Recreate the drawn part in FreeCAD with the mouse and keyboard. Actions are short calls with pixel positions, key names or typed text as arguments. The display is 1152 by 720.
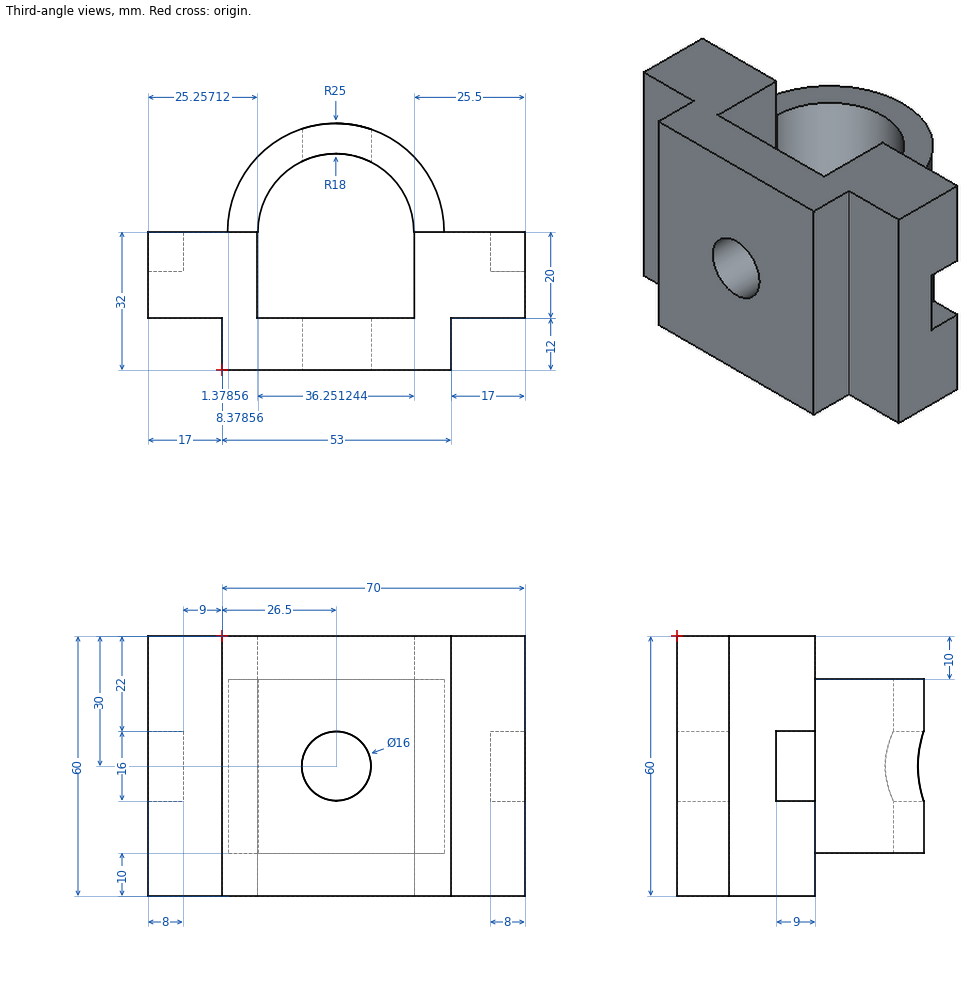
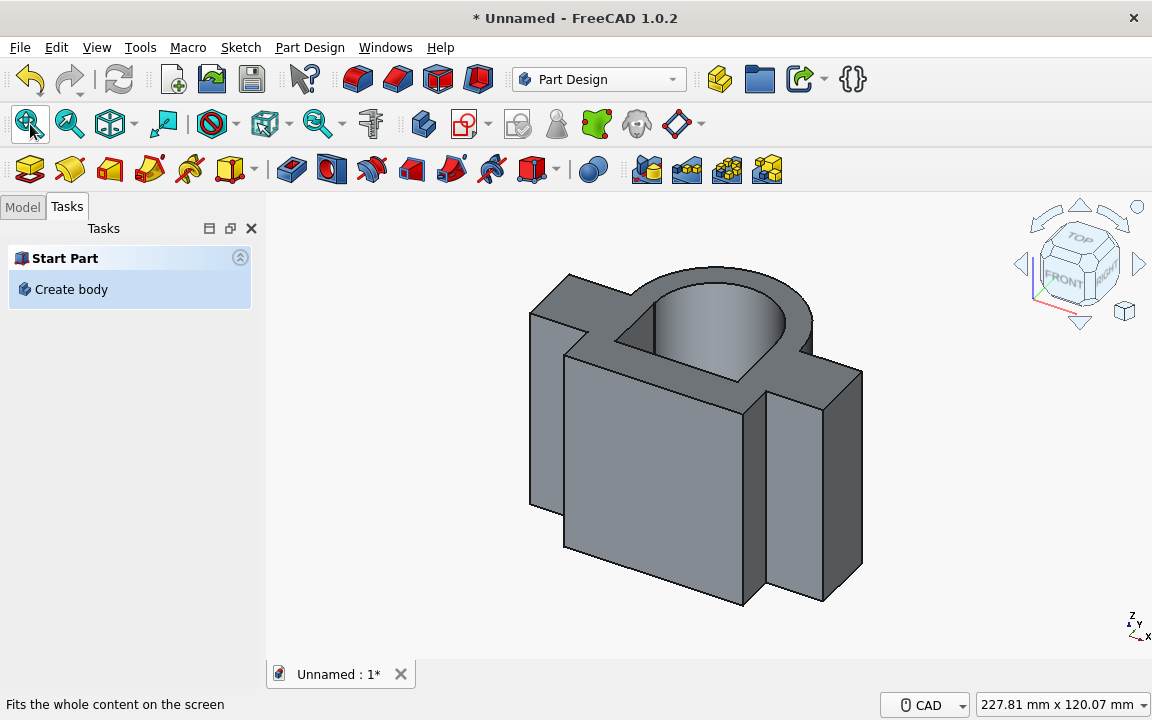
click(464, 124)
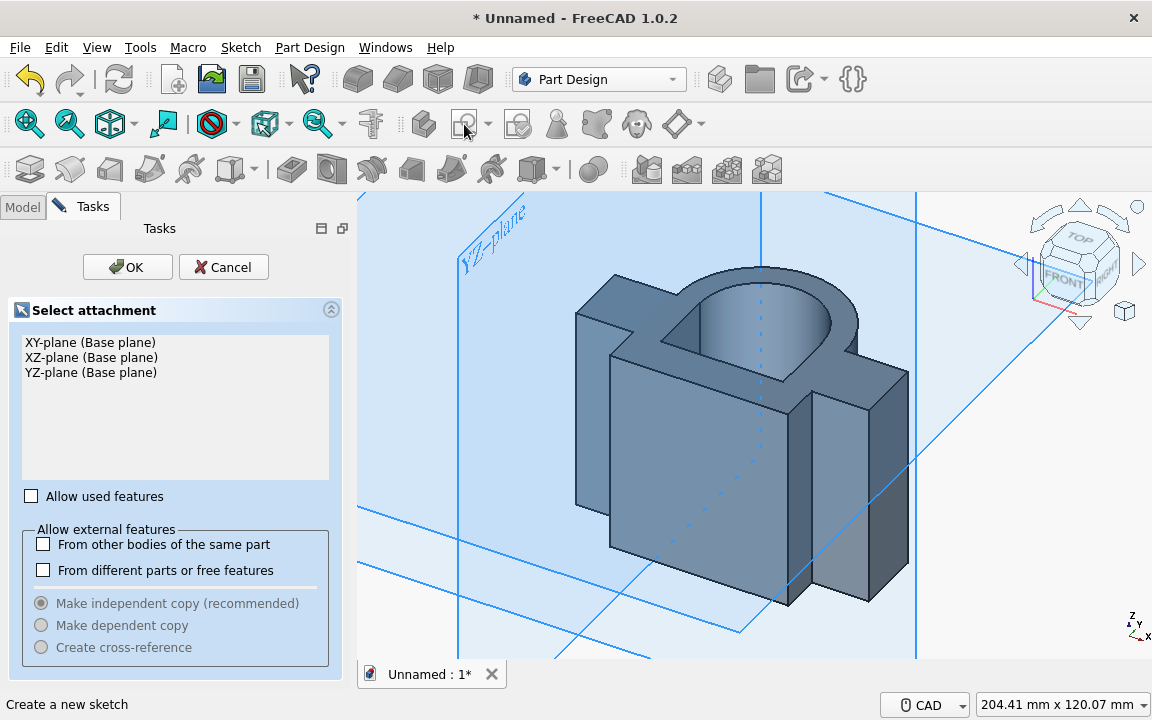
click(82, 342)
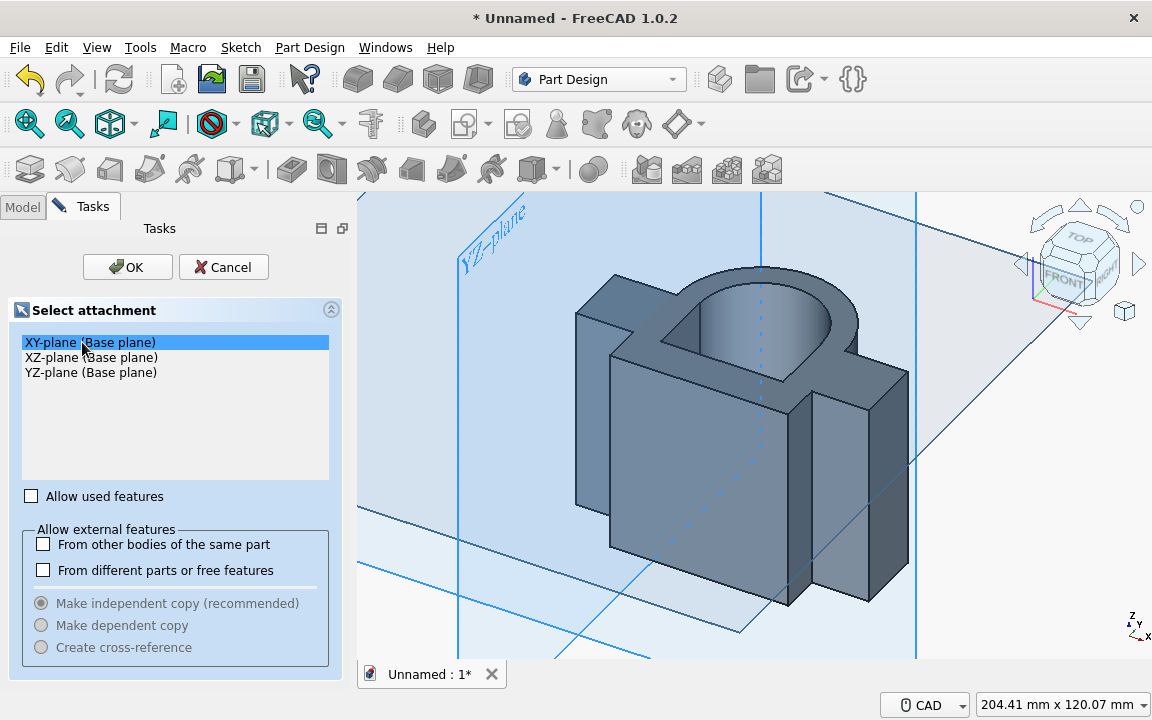
click(128, 267)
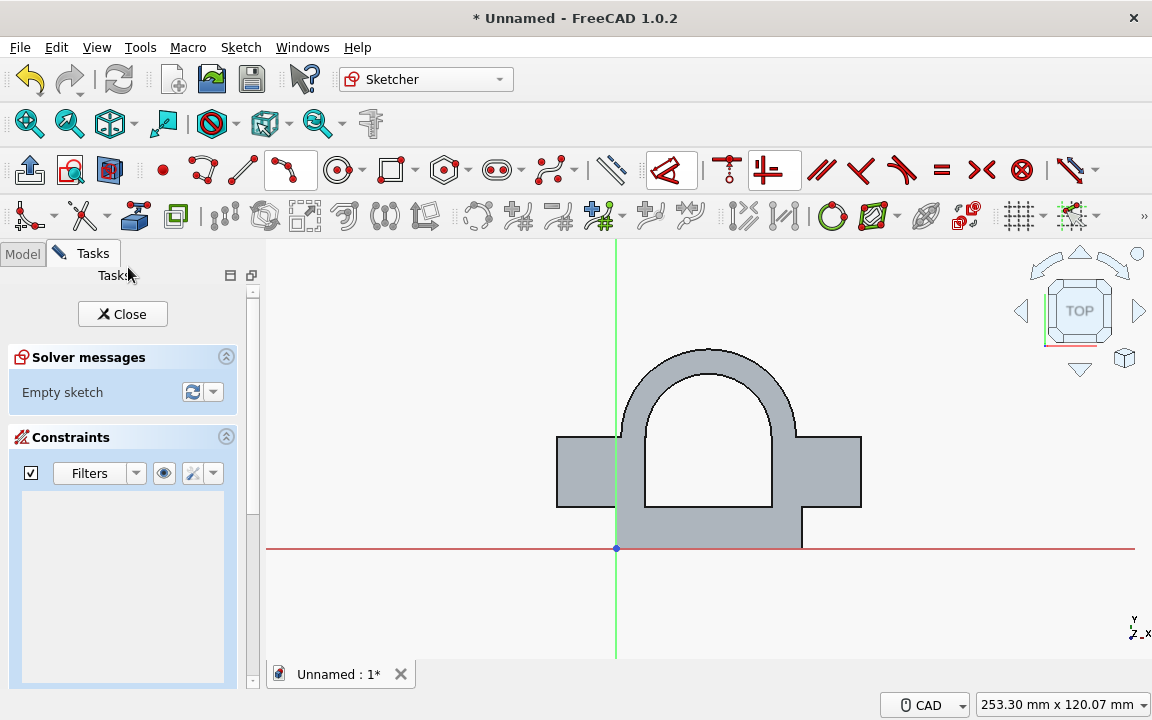
click(244, 170)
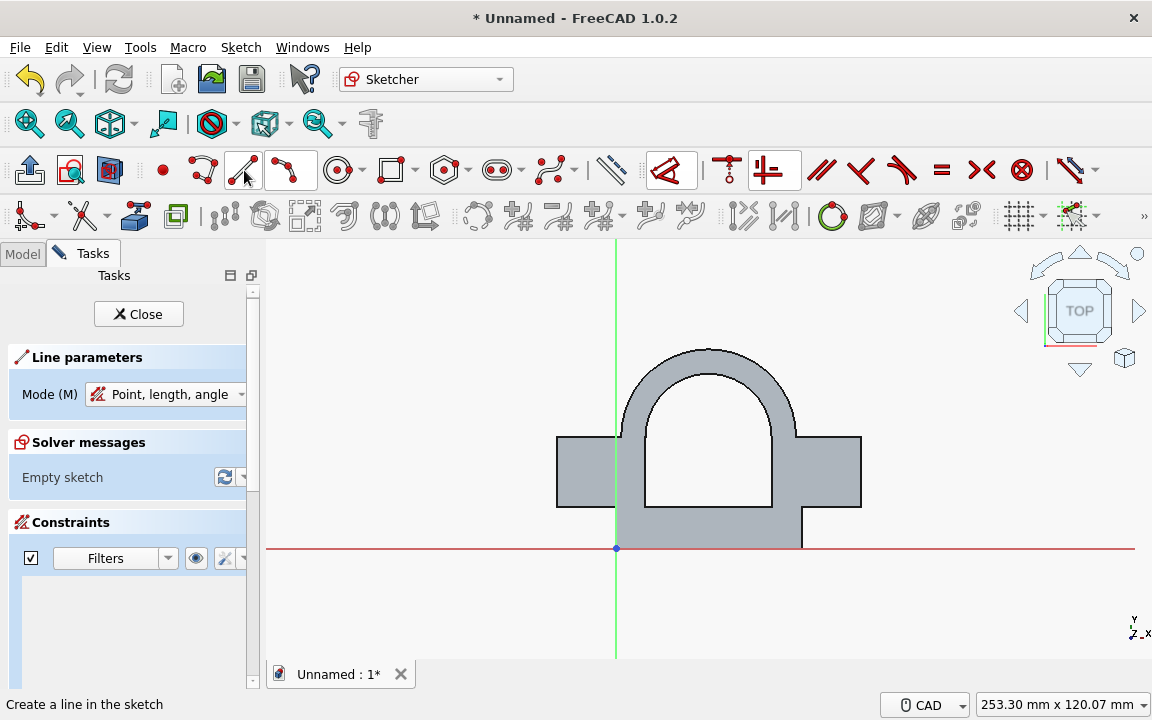
scroll(621, 437, up, 6)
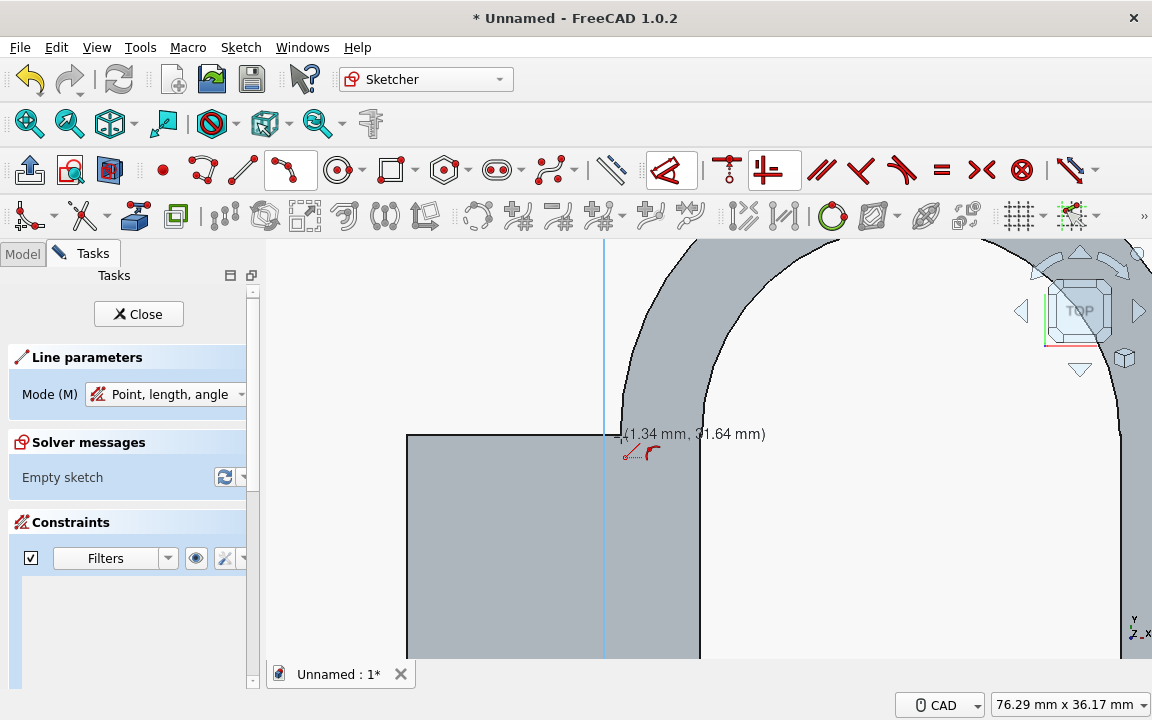
click(621, 435)
click(702, 435)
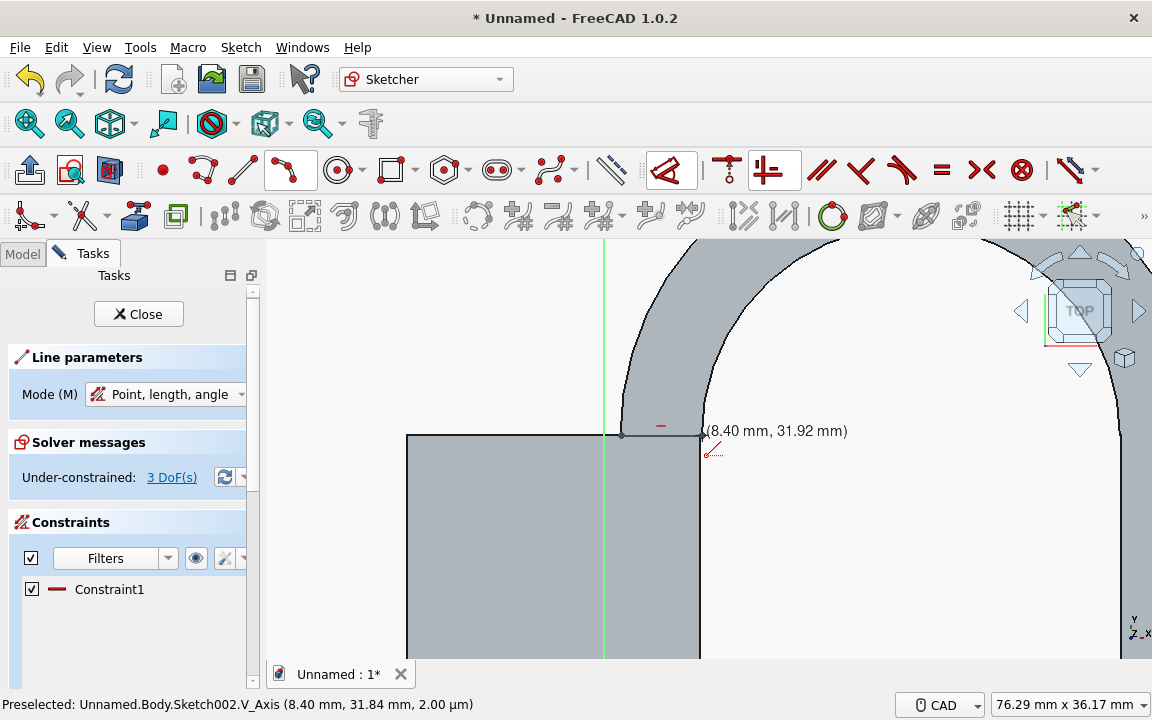
scroll(488, 433, down, 5)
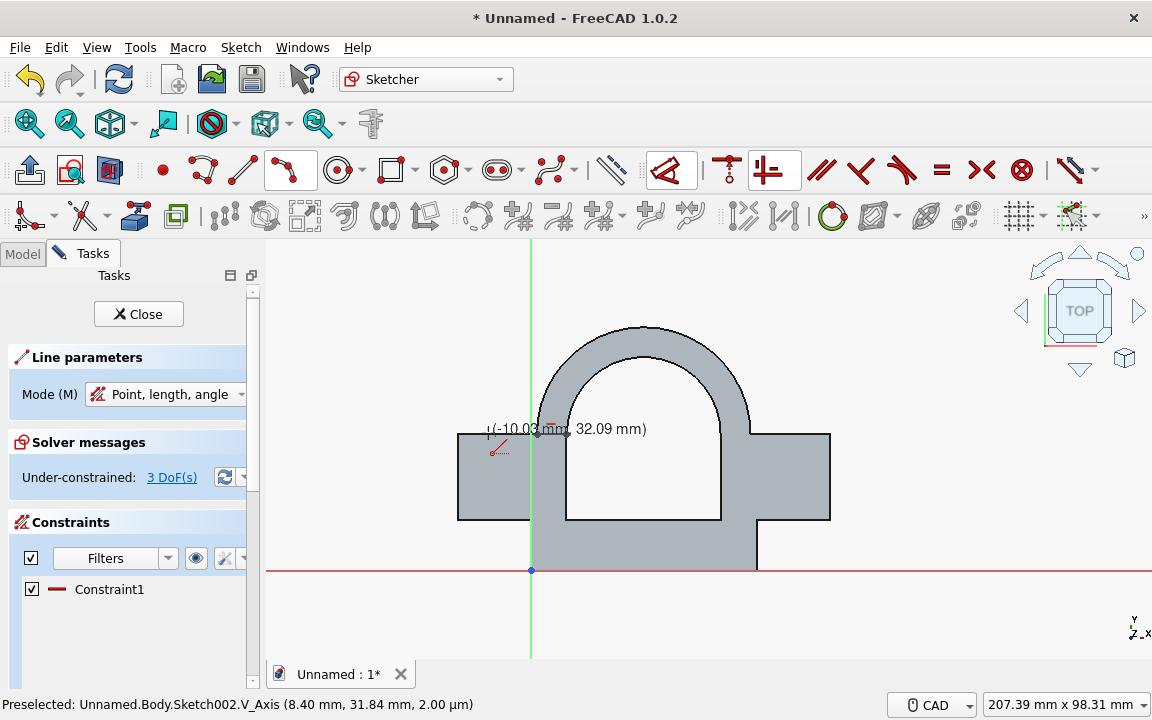
click(721, 434)
click(751, 434)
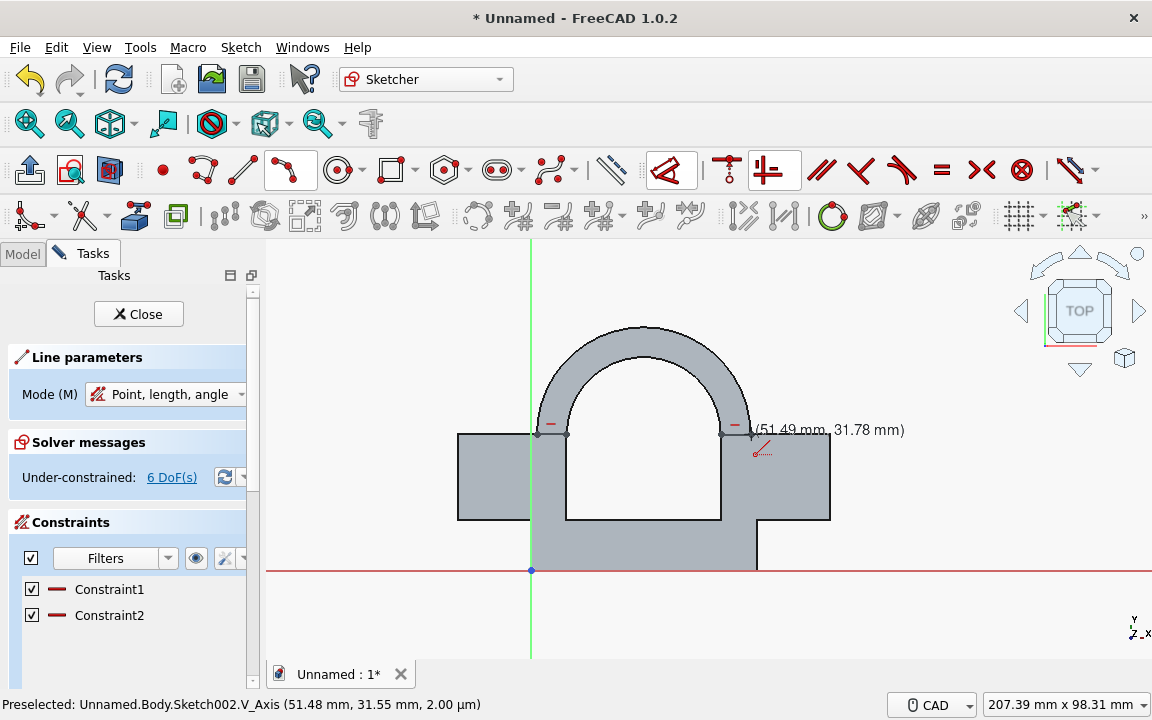
click(284, 170)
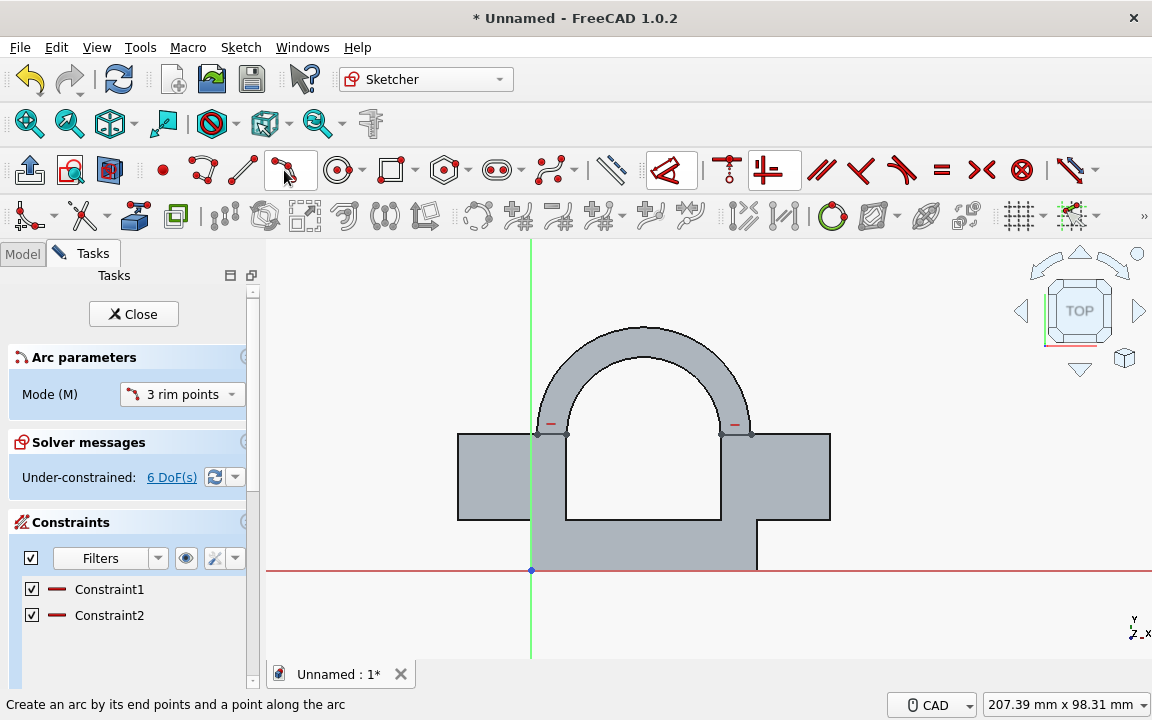
click(567, 434)
click(721, 435)
click(644, 357)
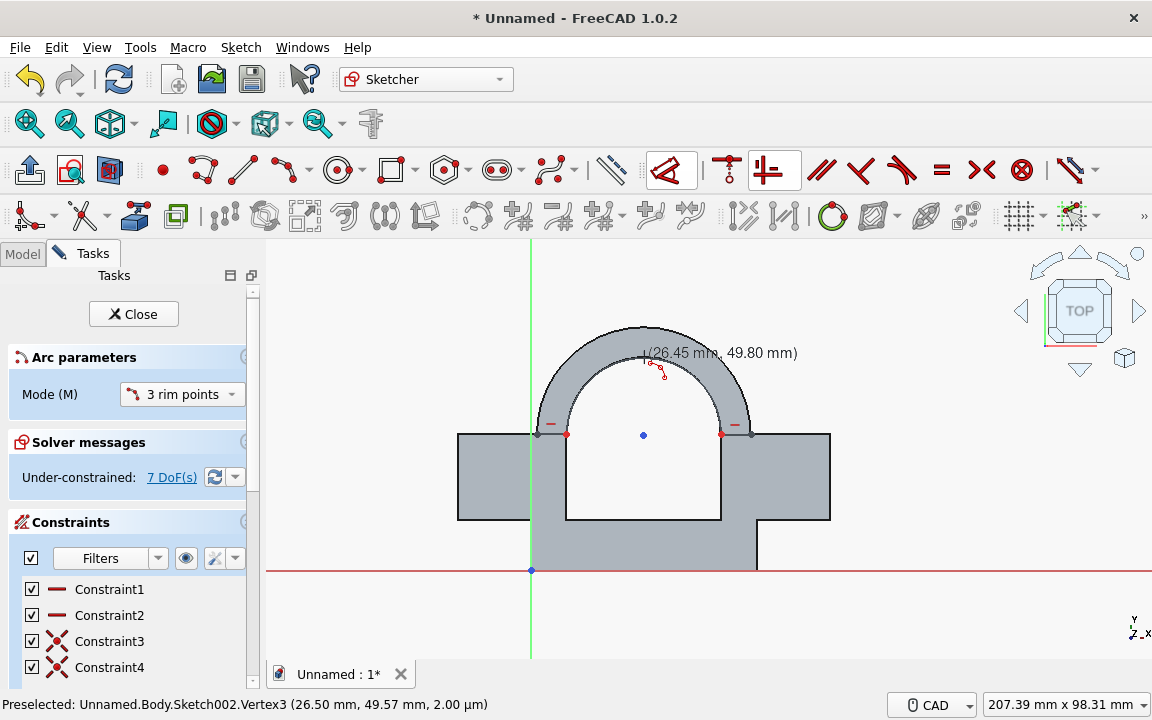
click(751, 435)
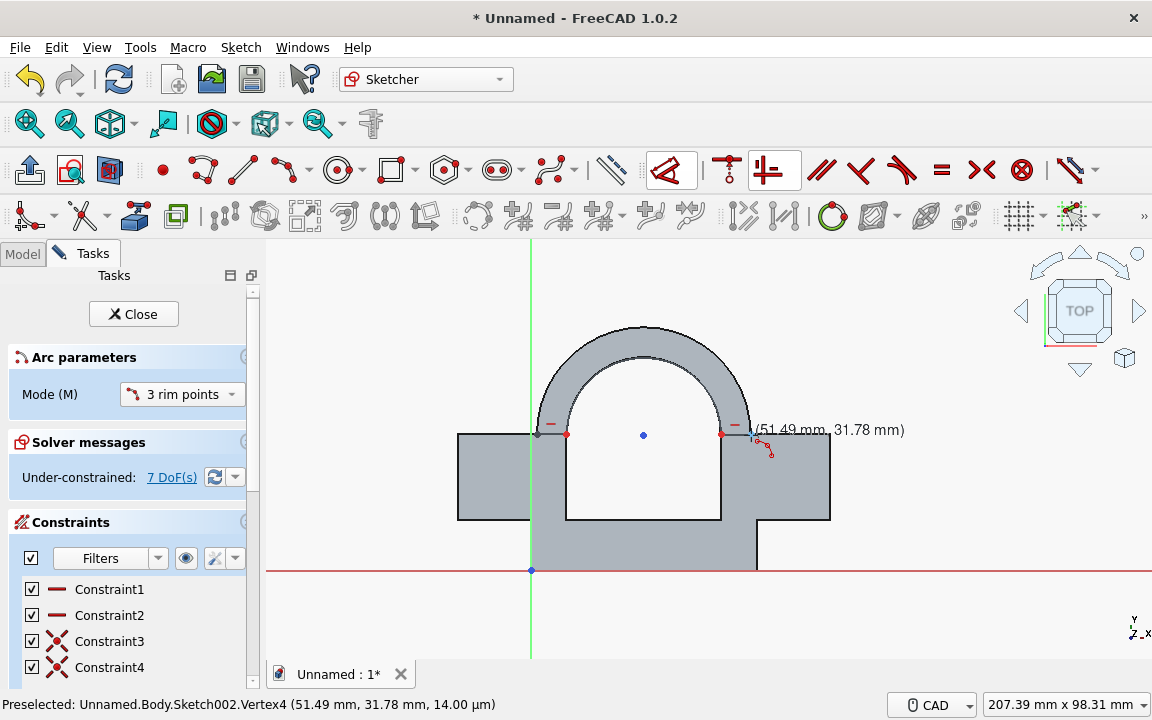
scroll(537, 434, up, 5)